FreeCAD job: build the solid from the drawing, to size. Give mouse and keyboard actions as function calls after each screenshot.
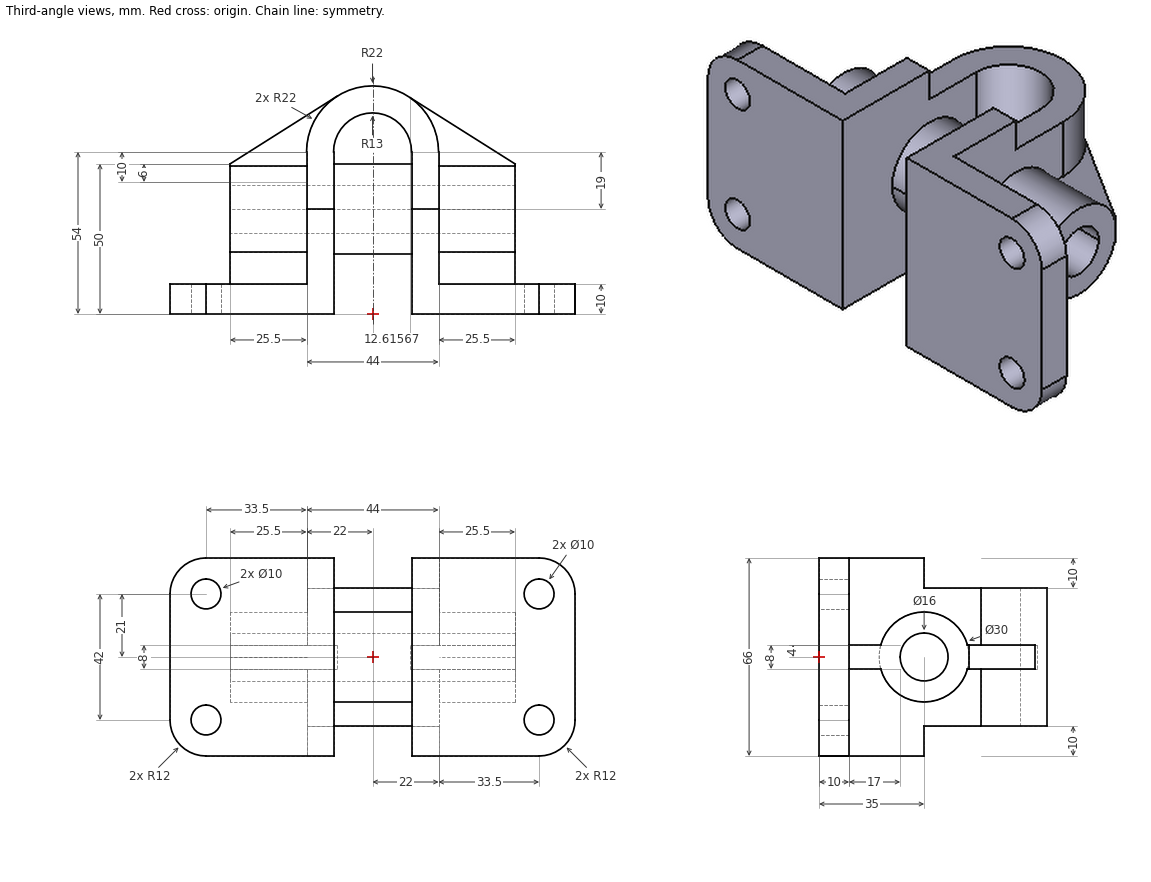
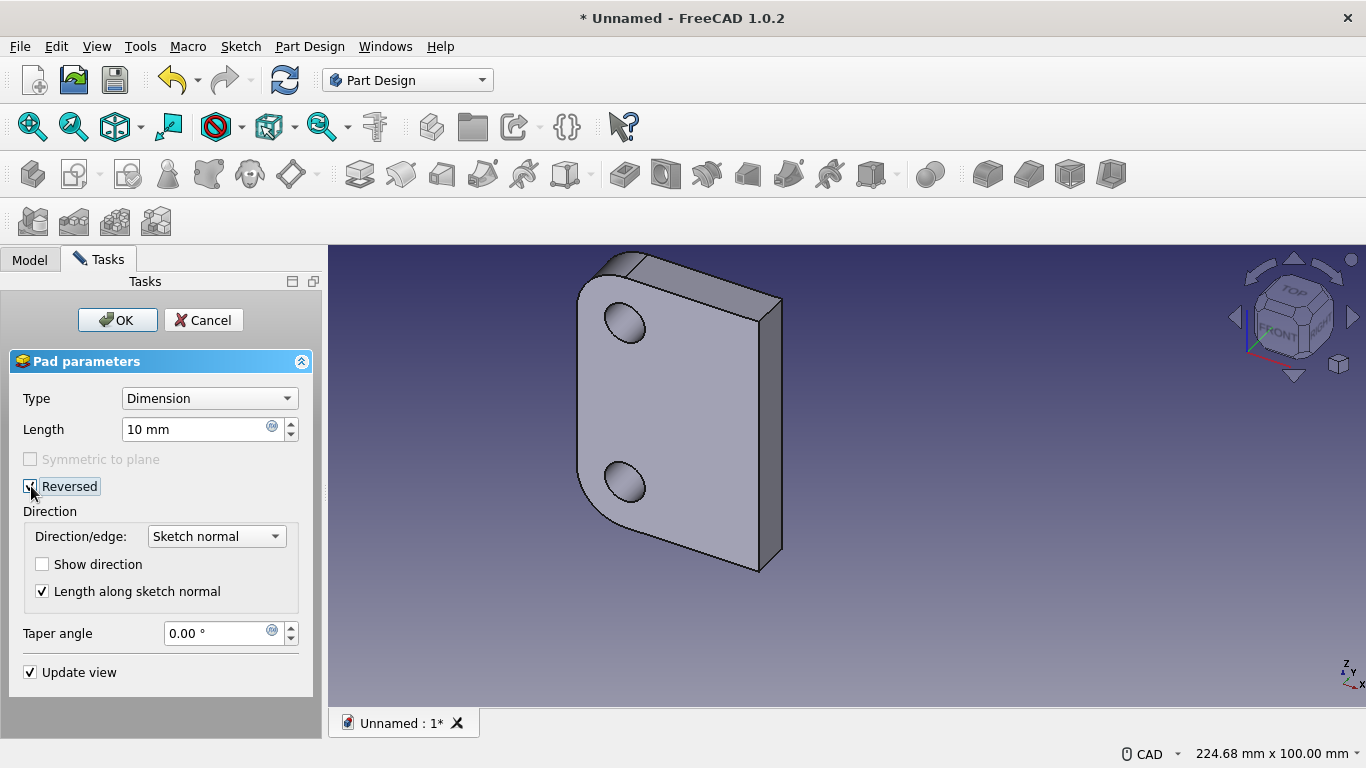
click(118, 320)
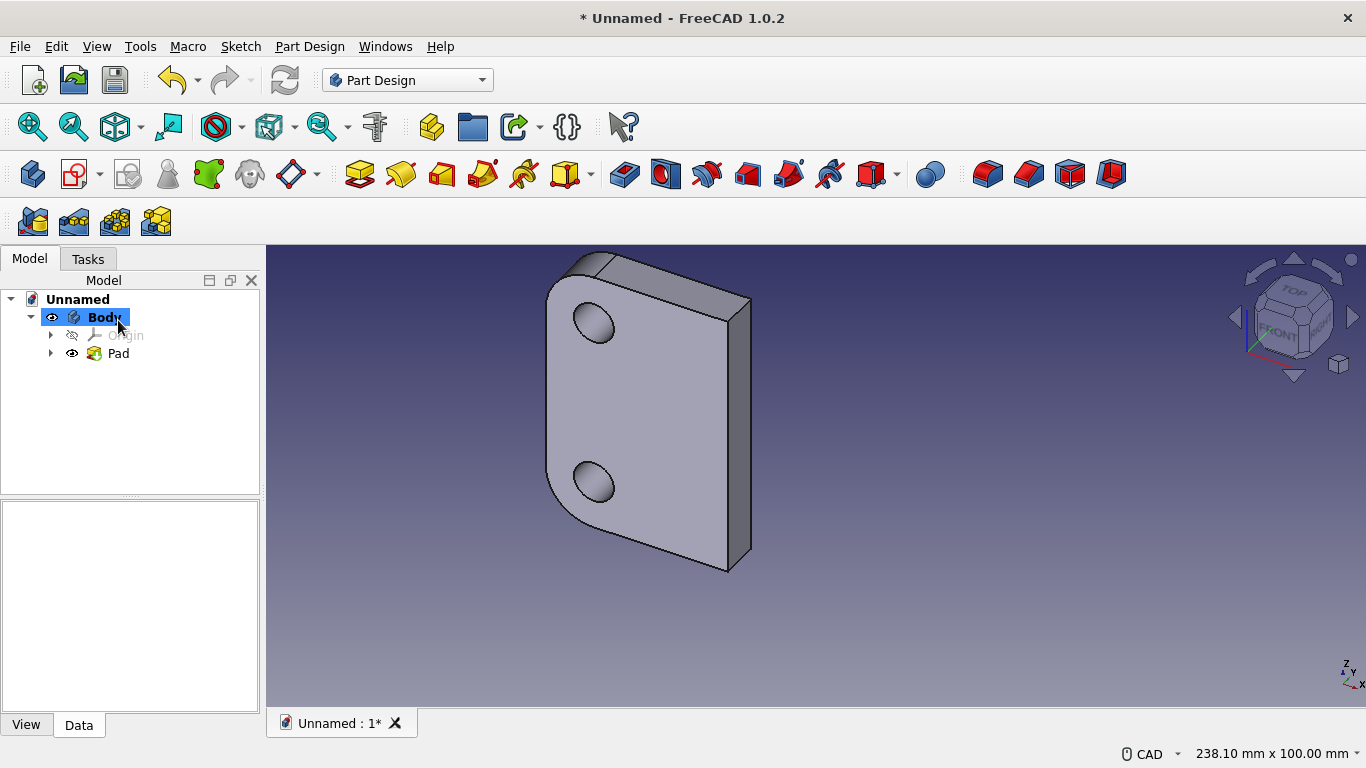
click(33, 128)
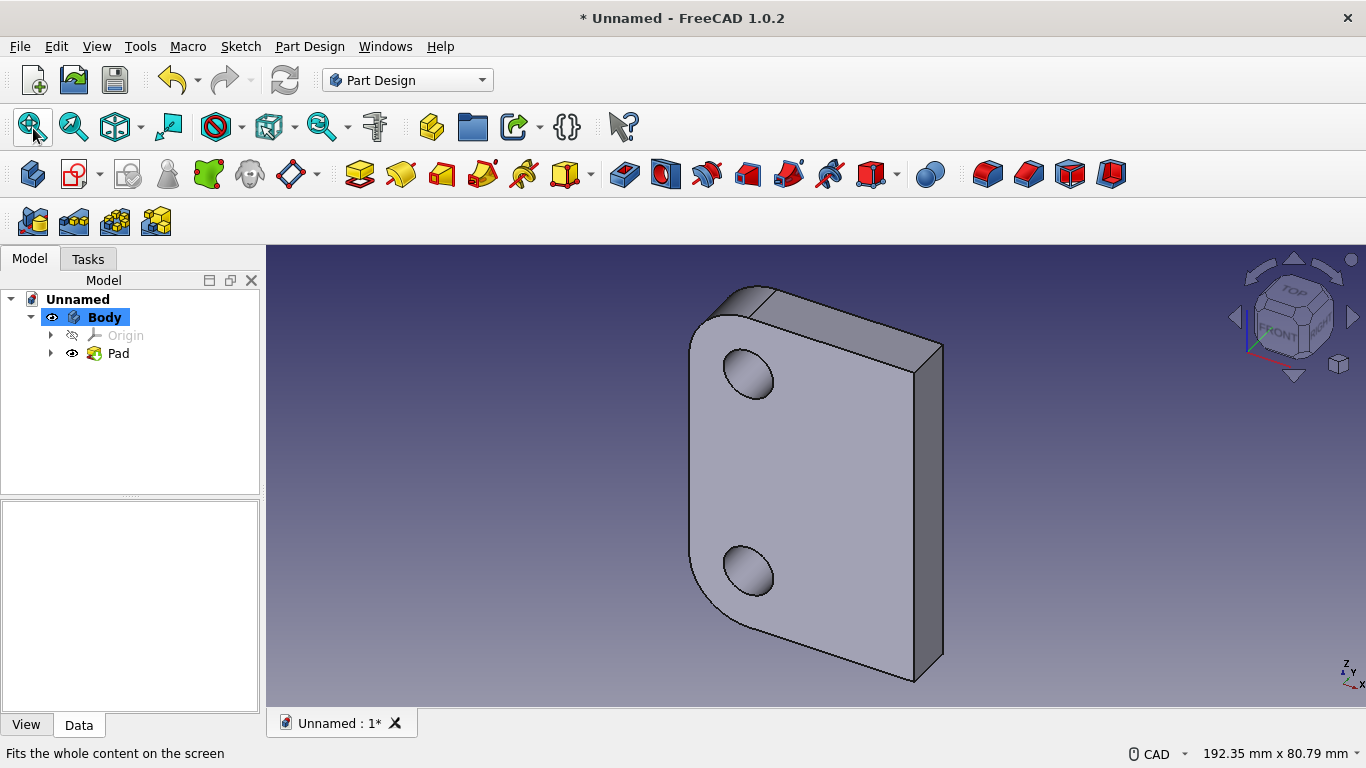
click(33, 174)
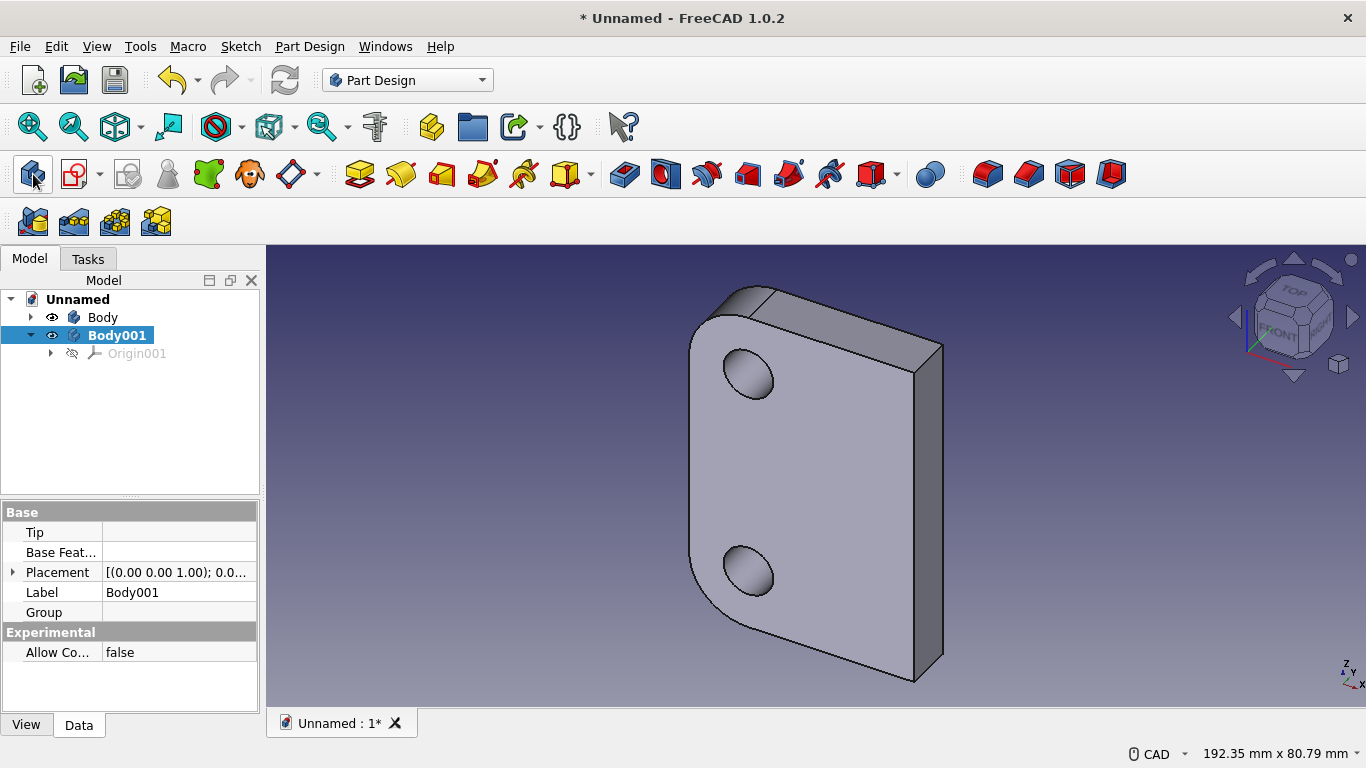
click(306, 667)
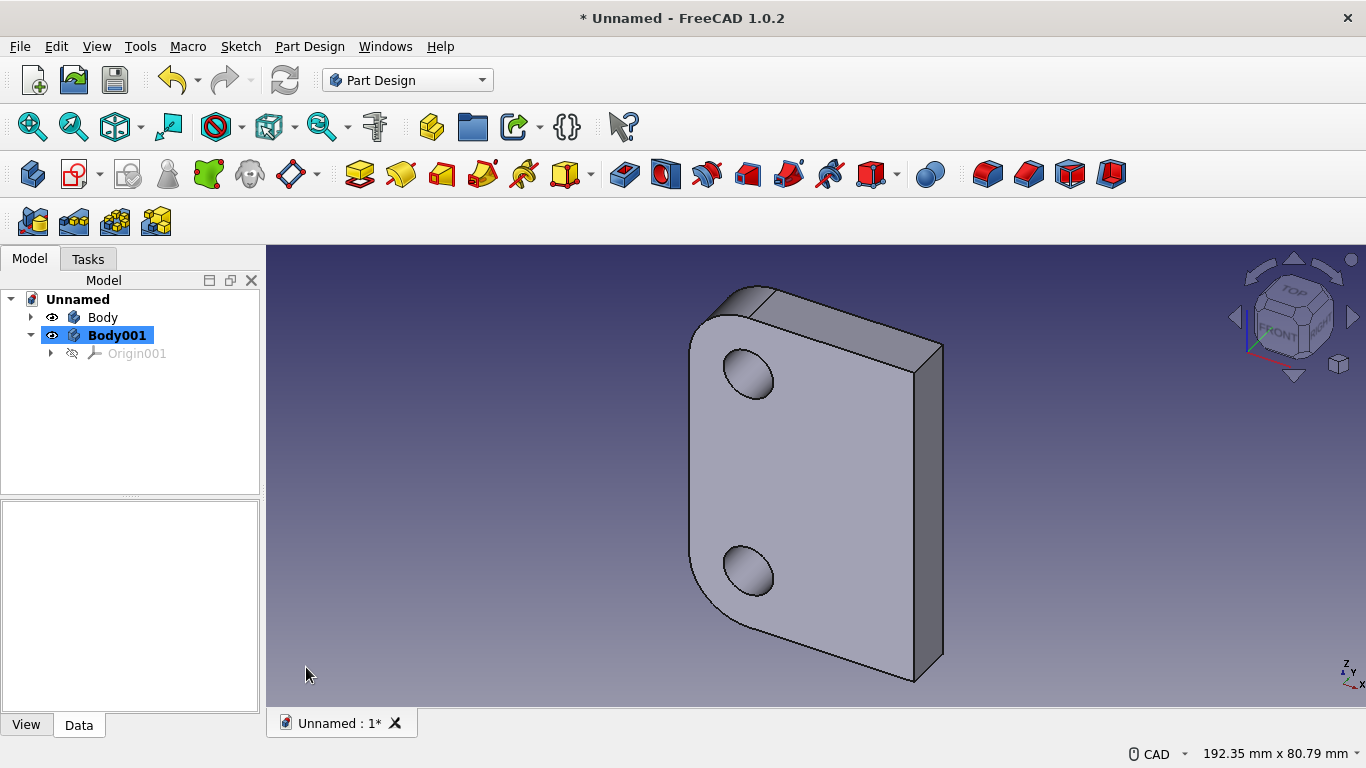
click(74, 174)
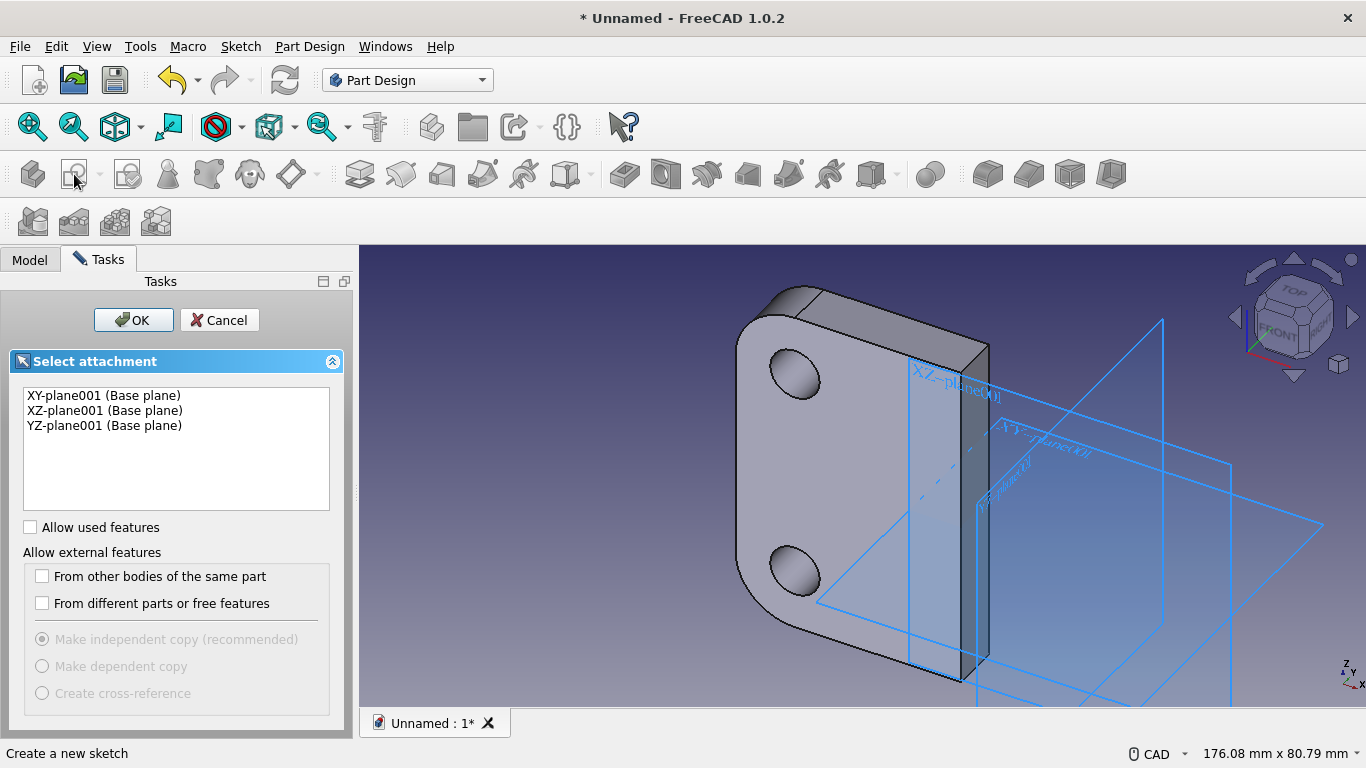
click(84, 410)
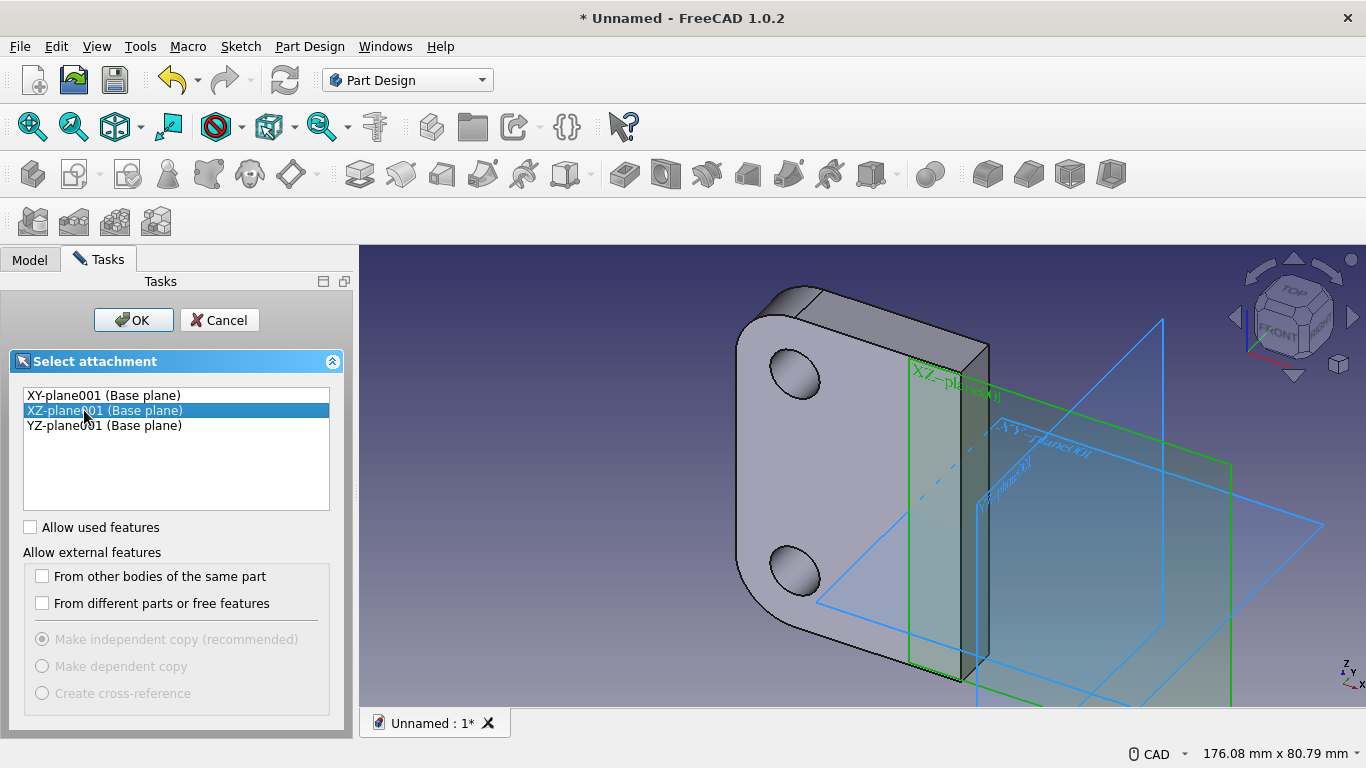
click(134, 320)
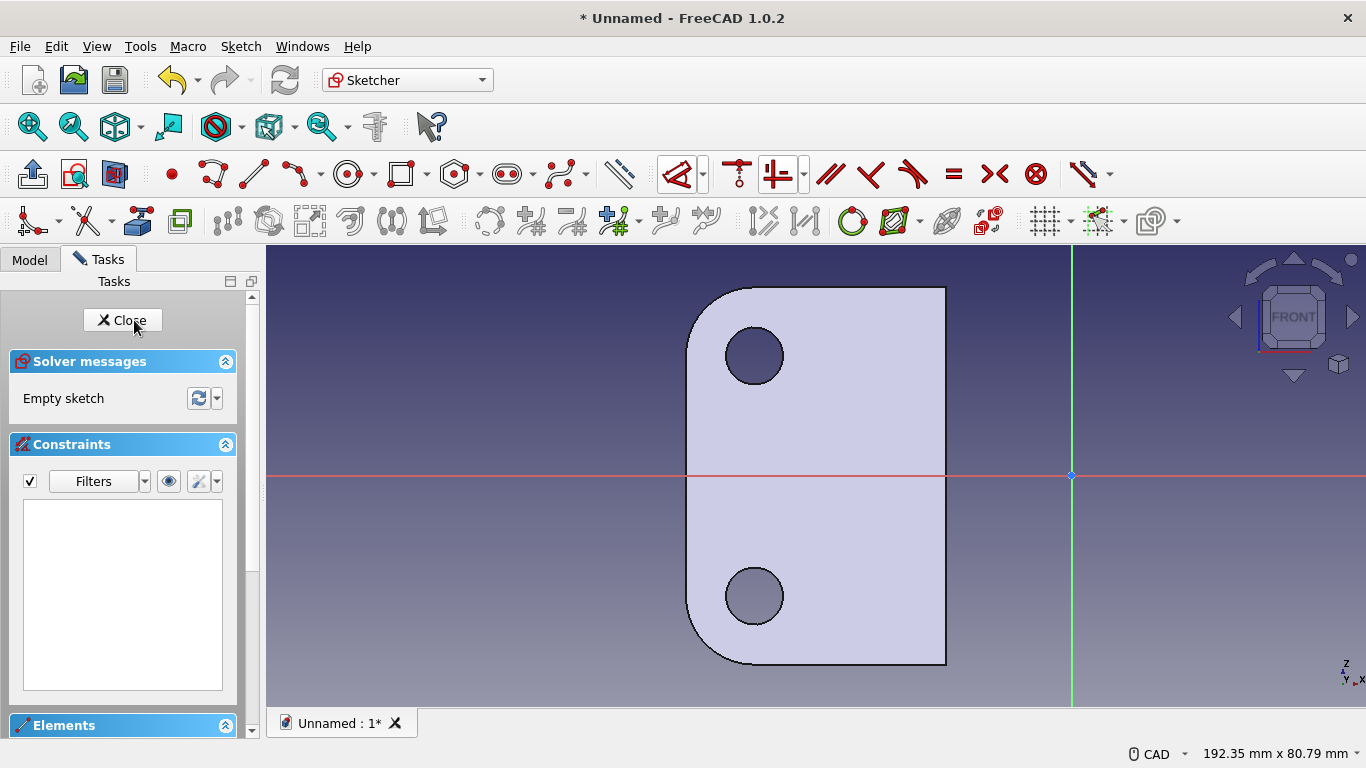
scroll(294, 476, down, 2)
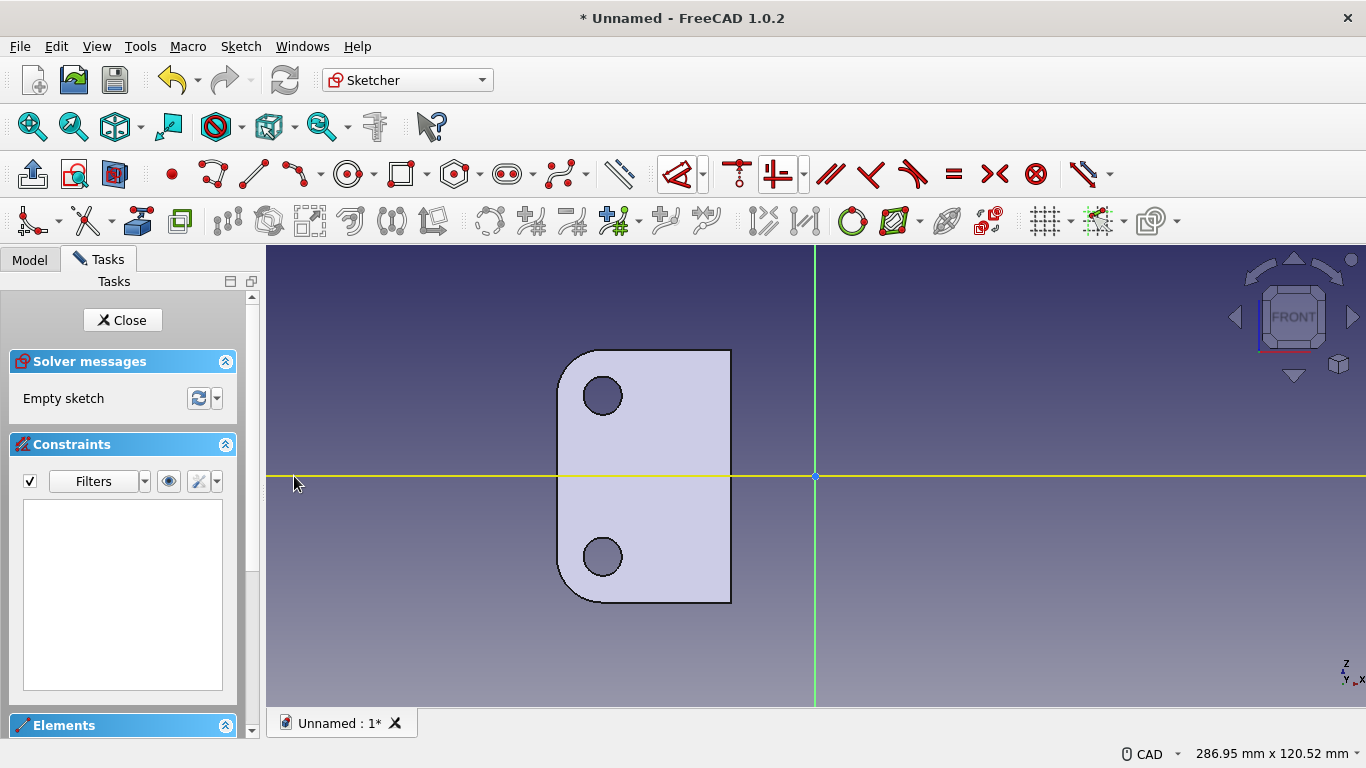
click(254, 174)